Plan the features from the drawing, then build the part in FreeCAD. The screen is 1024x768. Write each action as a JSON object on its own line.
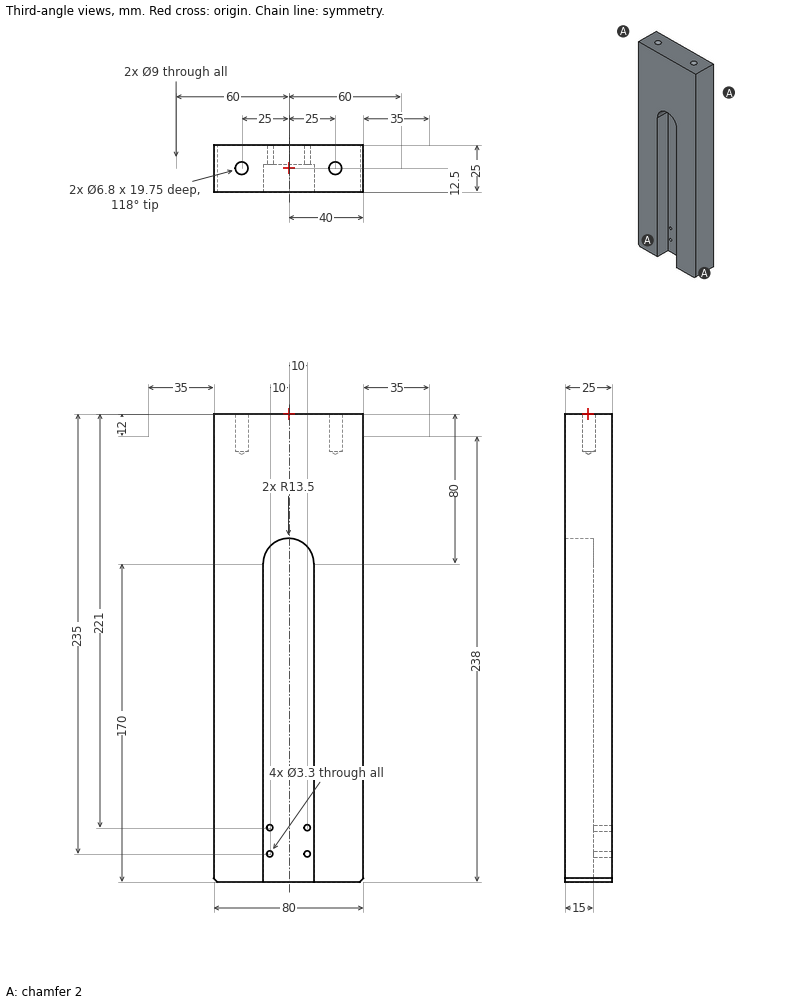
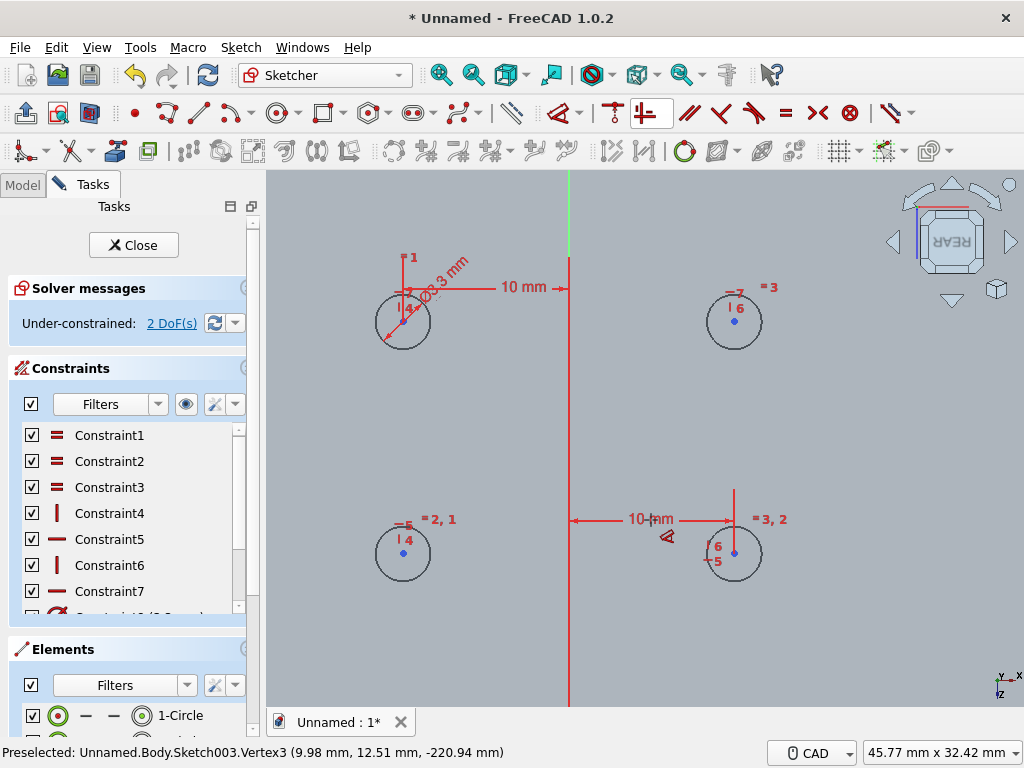
{"action": "left_click", "coordinate": [403, 322]}
{"action": "left_click", "coordinate": [369, 501]}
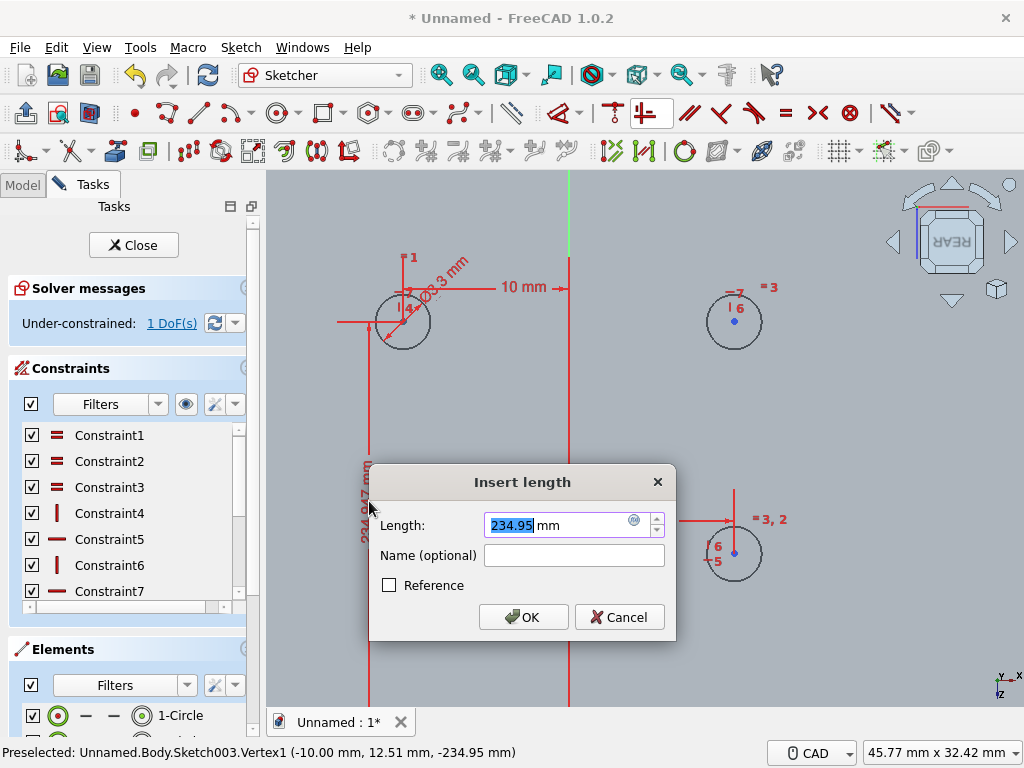
{"action": "type", "text": "235"}
{"action": "key", "text": "Return"}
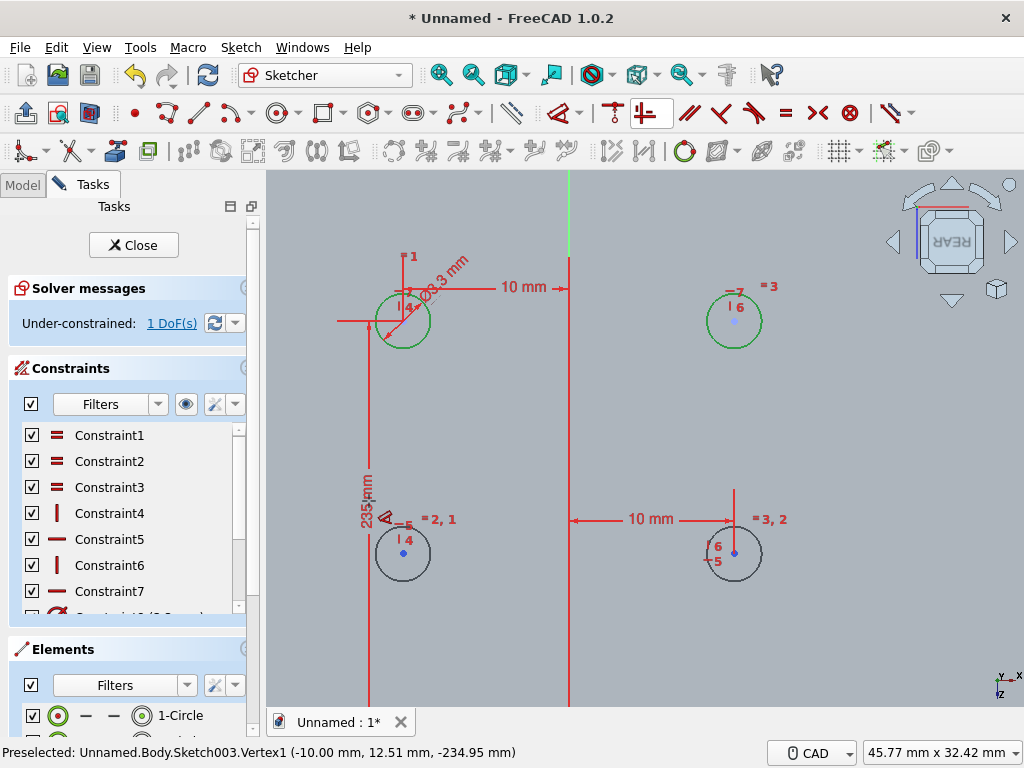
{"action": "left_click", "coordinate": [403, 554]}
{"action": "left_click", "coordinate": [369, 616]}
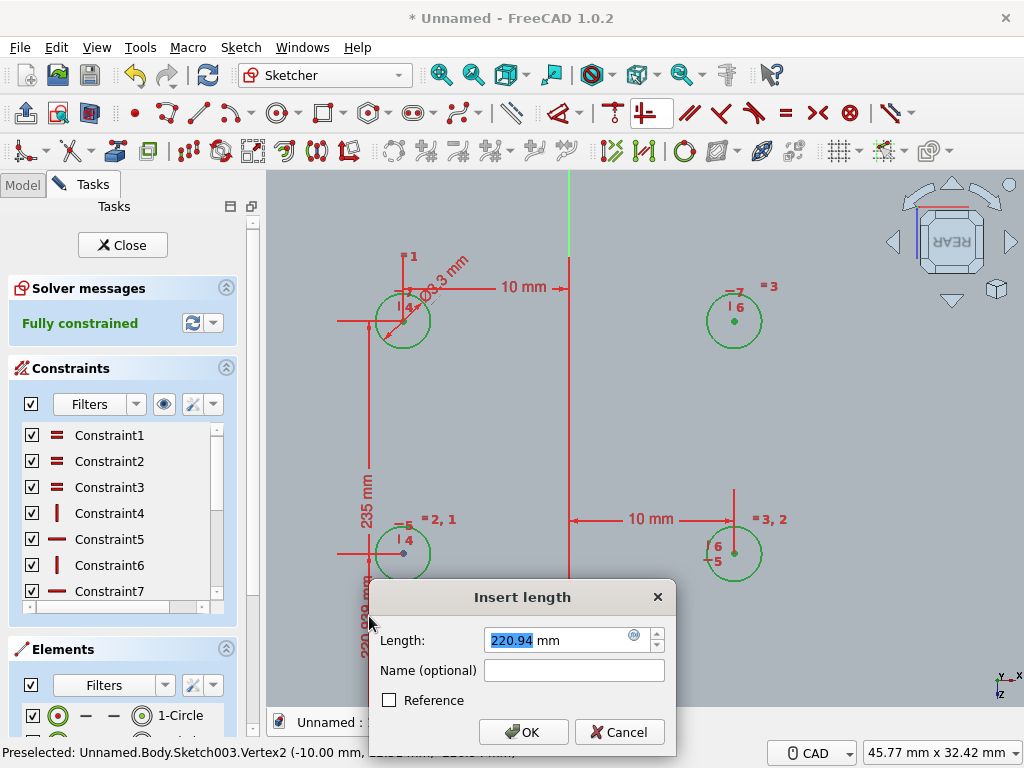
{"action": "type", "text": "221"}
{"action": "key", "text": "Return"}
{"action": "key", "text": "Escape"}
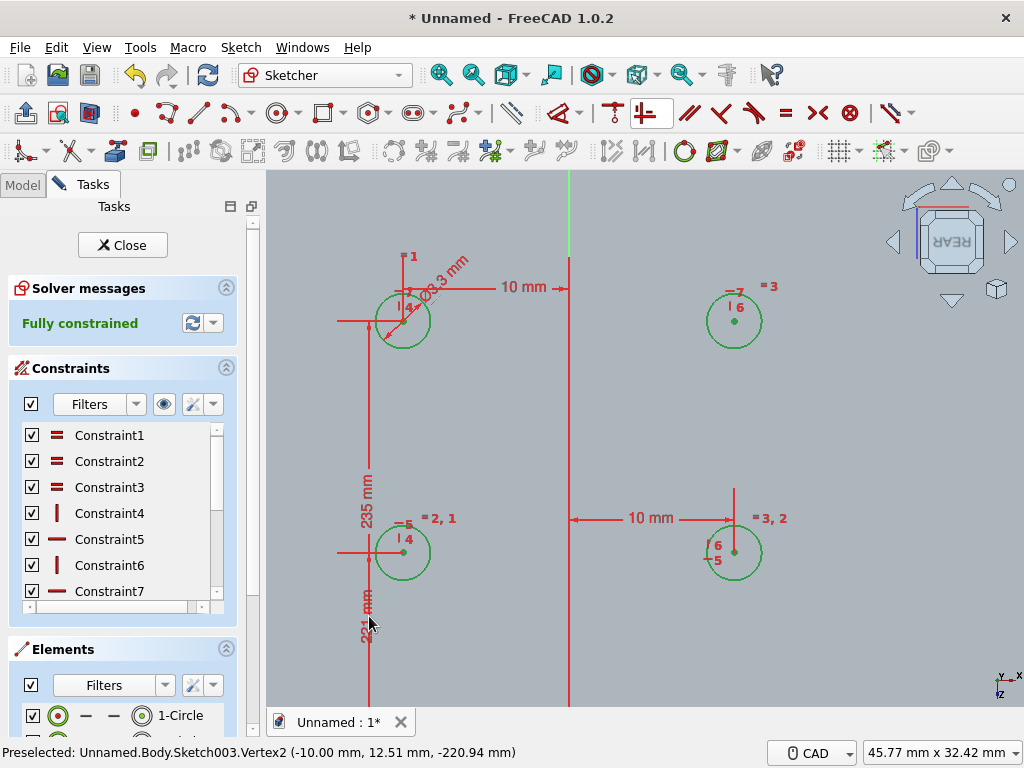
{"action": "left_click", "coordinate": [123, 245]}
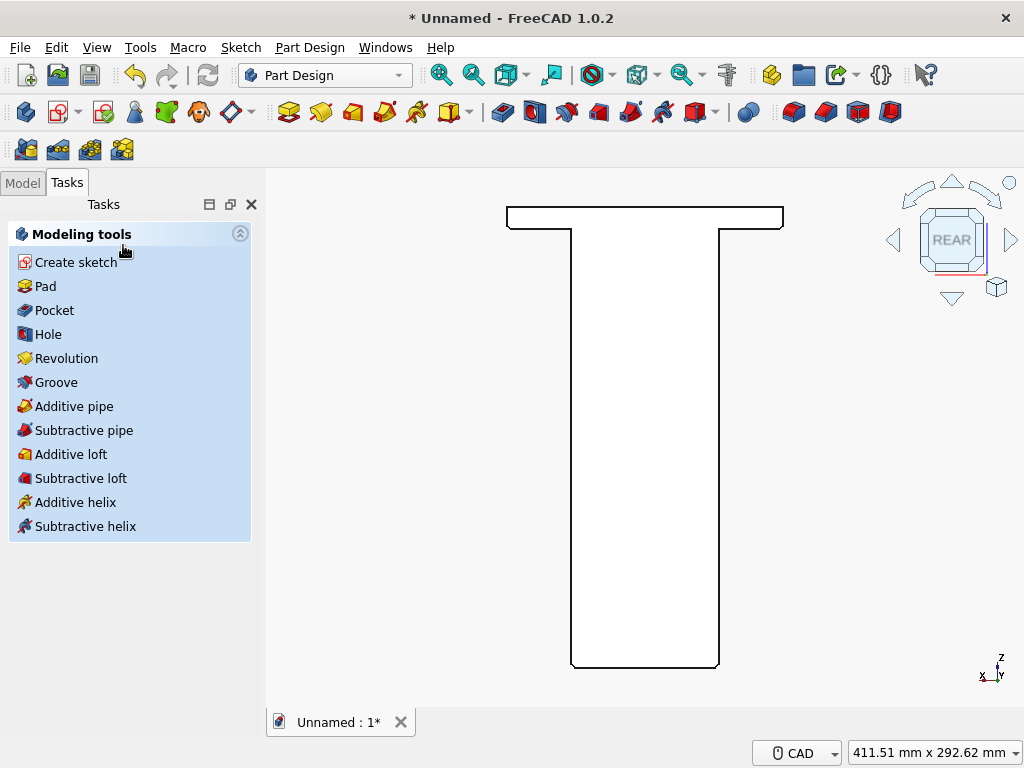
{"action": "left_click", "coordinate": [536, 112]}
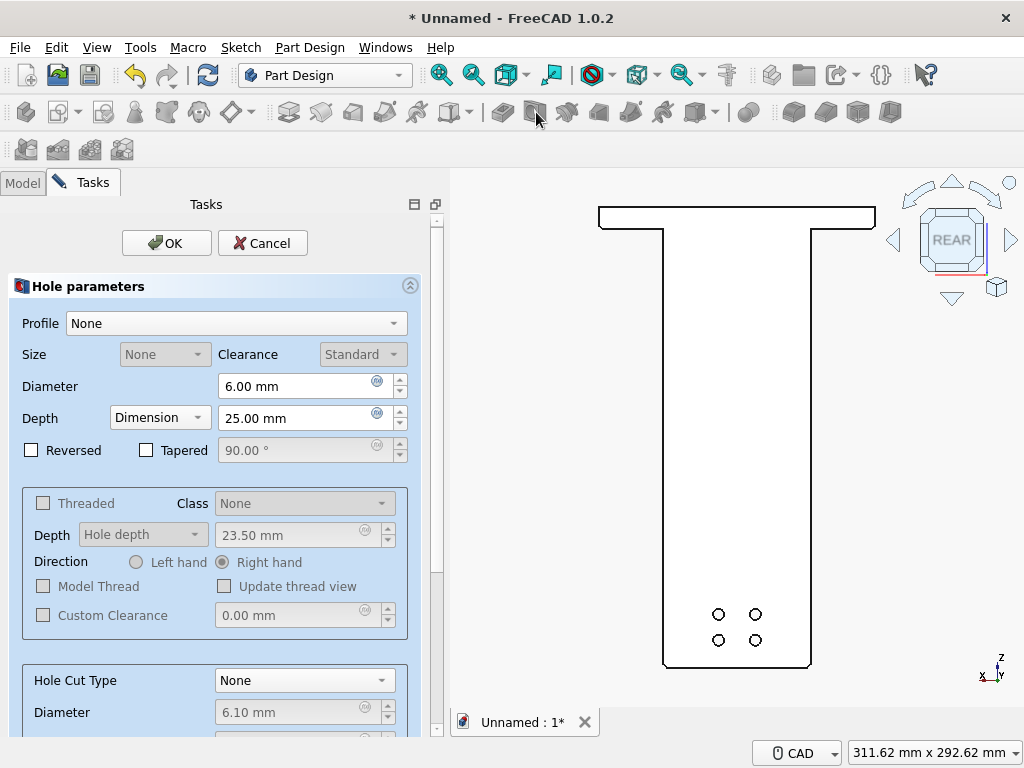
{"action": "triple_click", "coordinate": [305, 386]}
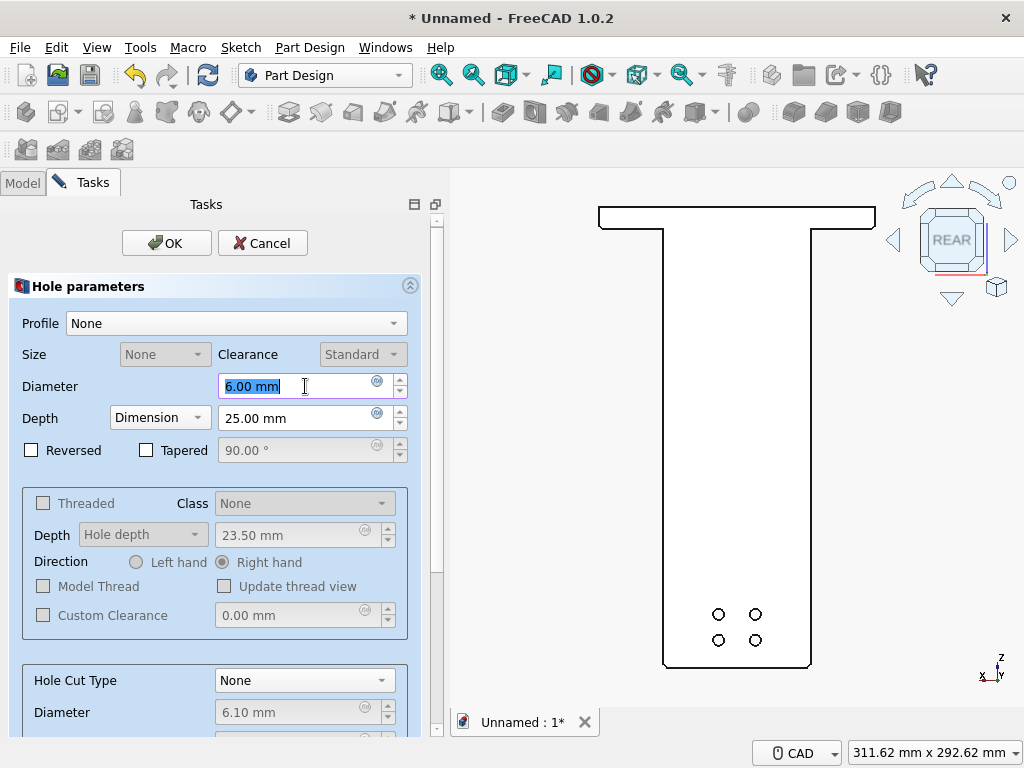
{"action": "type", "text": "3.3"}
{"action": "key", "text": "Tab"}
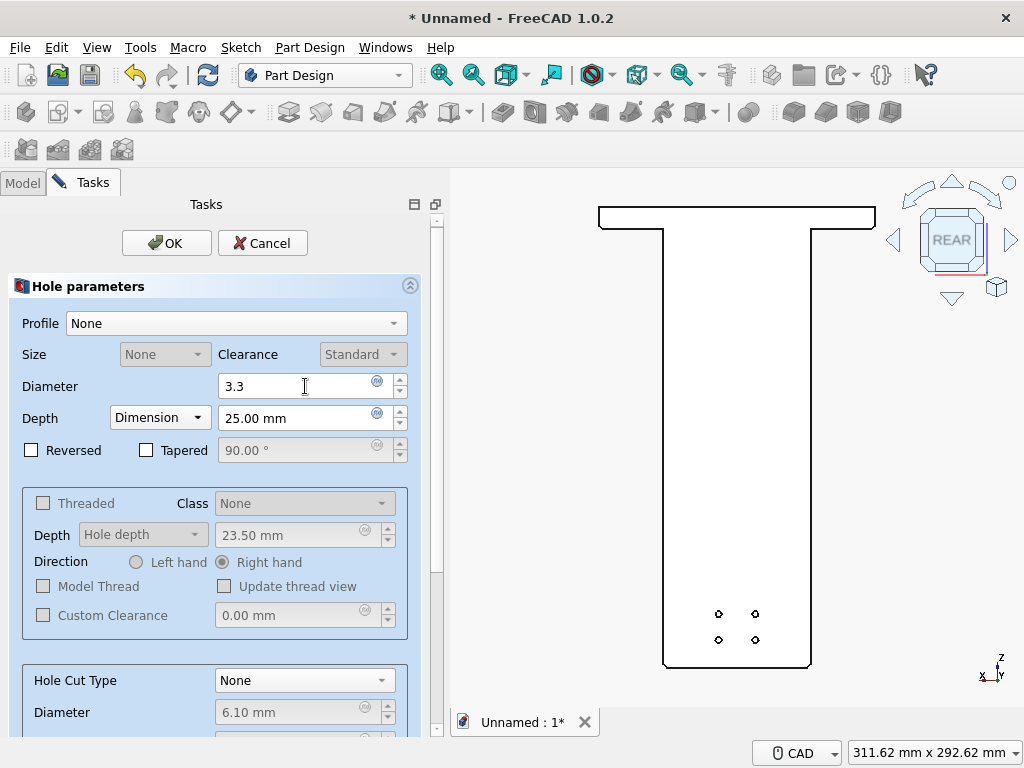
{"action": "left_click", "coordinate": [161, 418]}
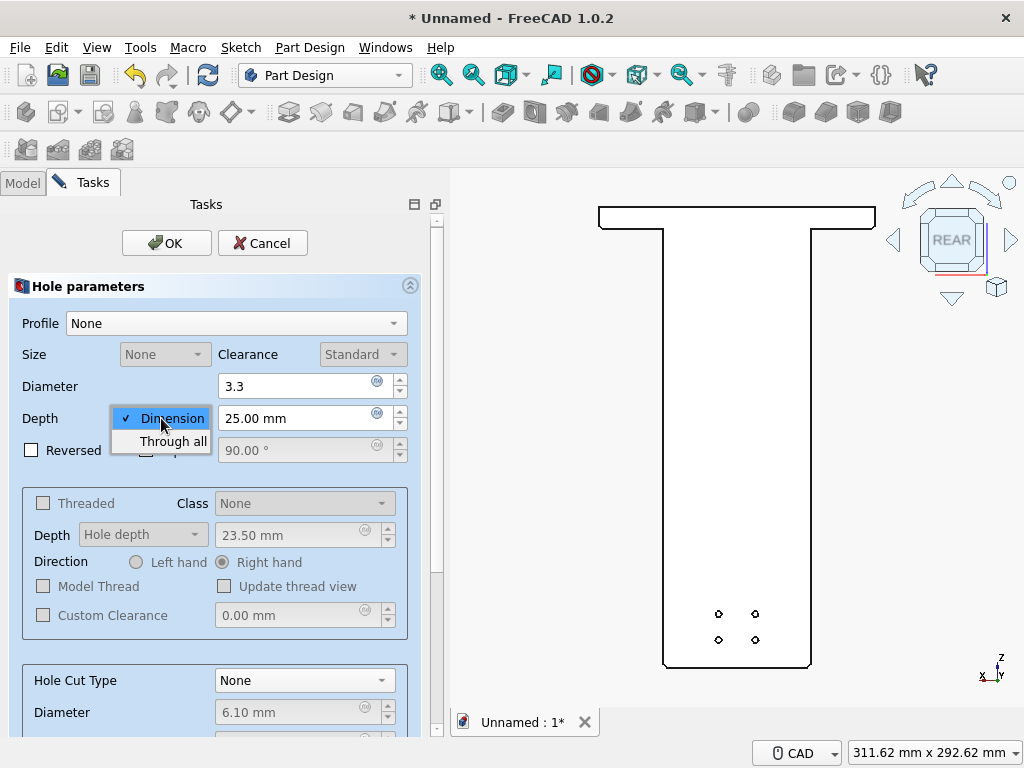
{"action": "left_click", "coordinate": [160, 442]}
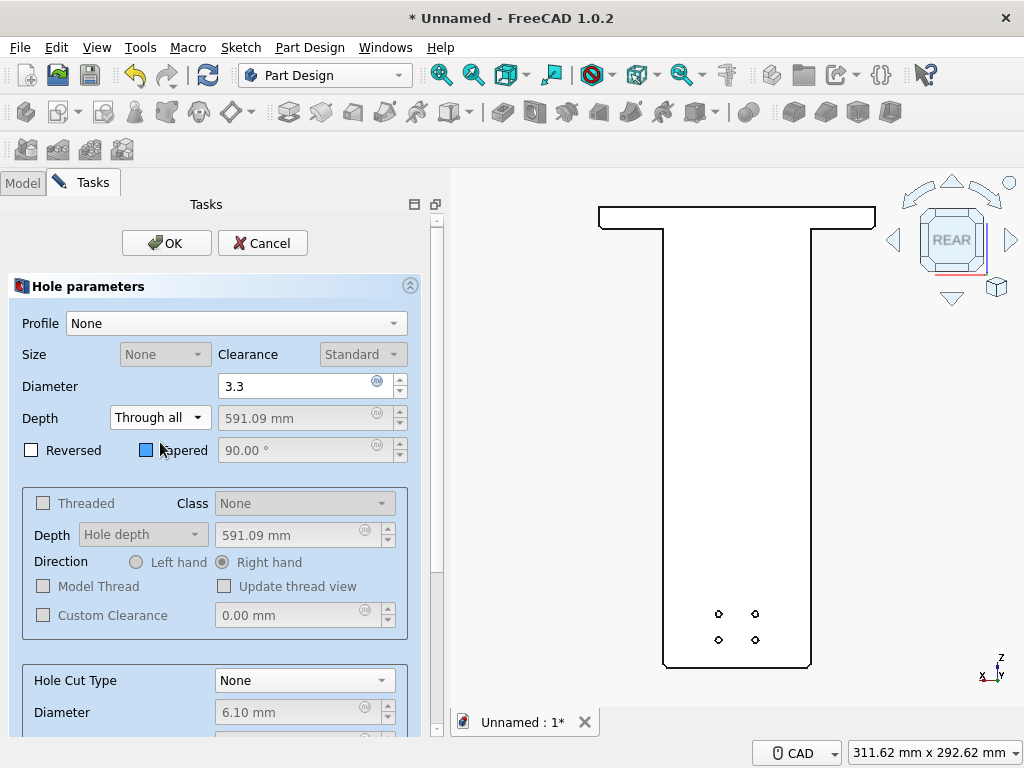
{"action": "left_click", "coordinate": [167, 243]}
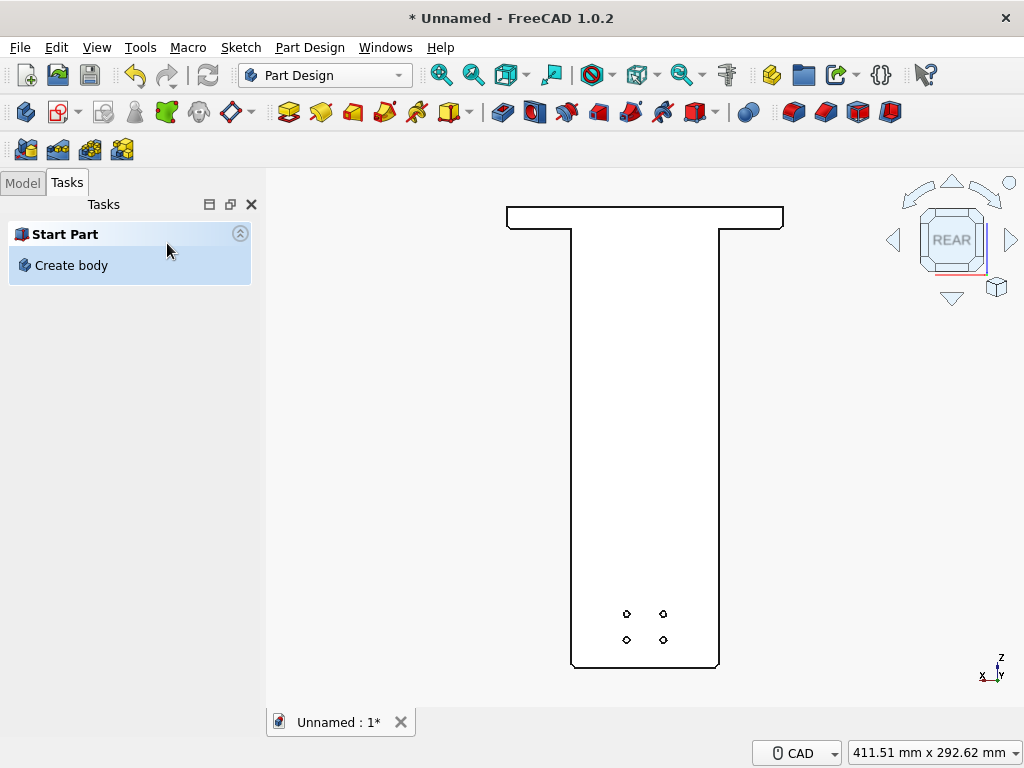
{"action": "key", "text": "5"}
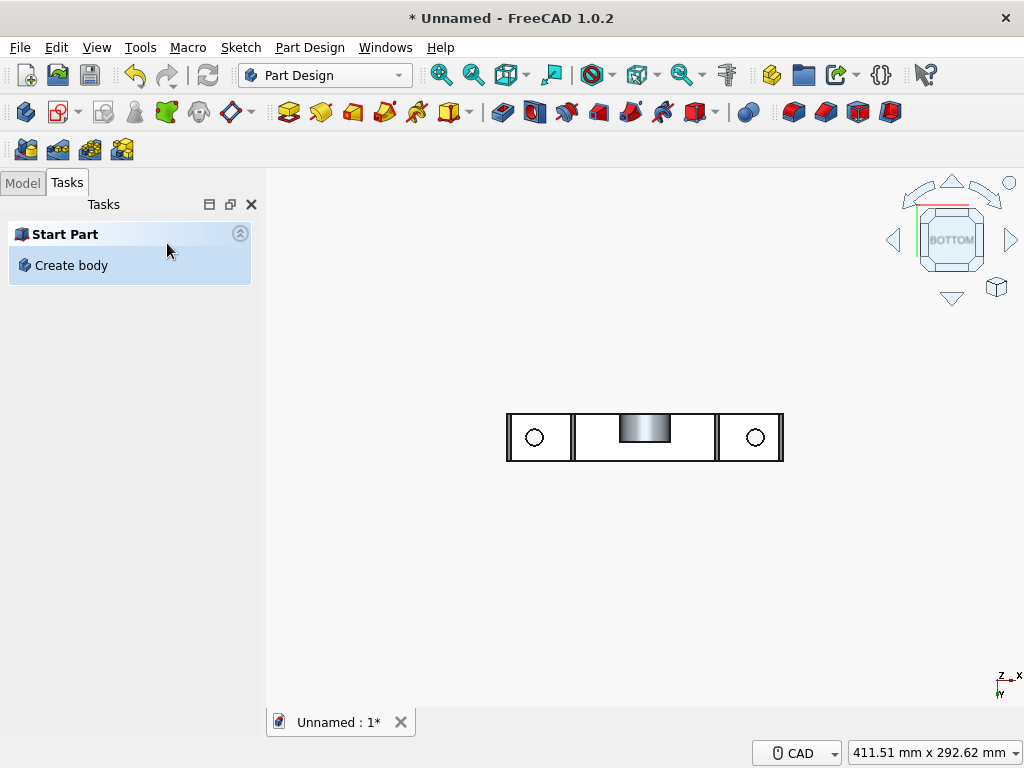
{"action": "left_click", "coordinate": [442, 76]}